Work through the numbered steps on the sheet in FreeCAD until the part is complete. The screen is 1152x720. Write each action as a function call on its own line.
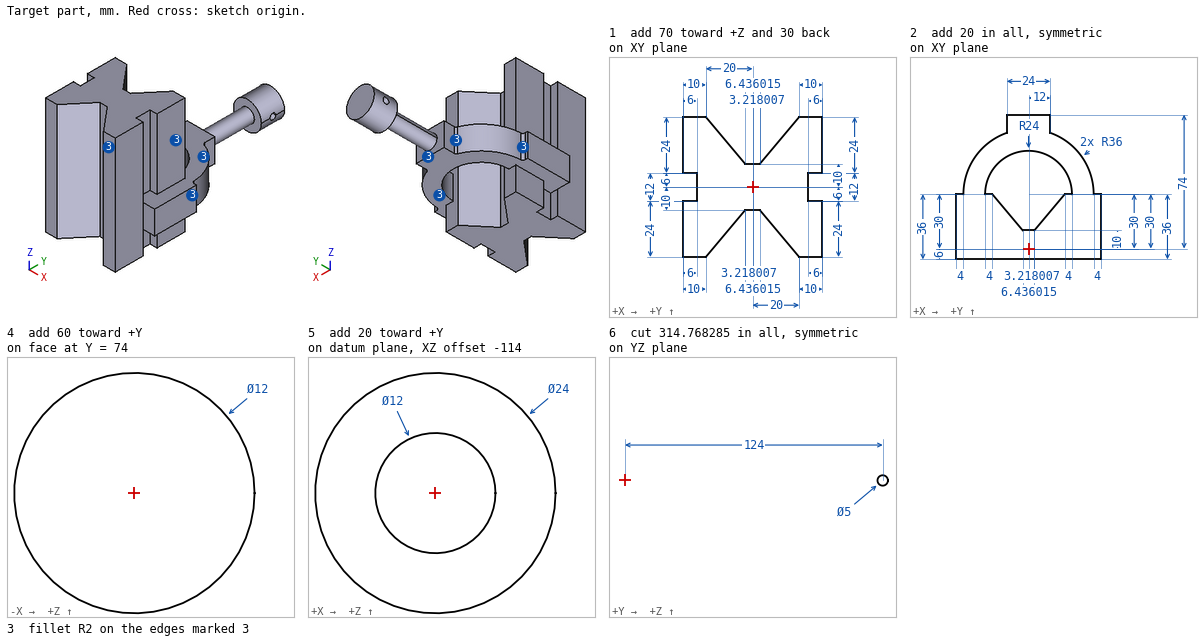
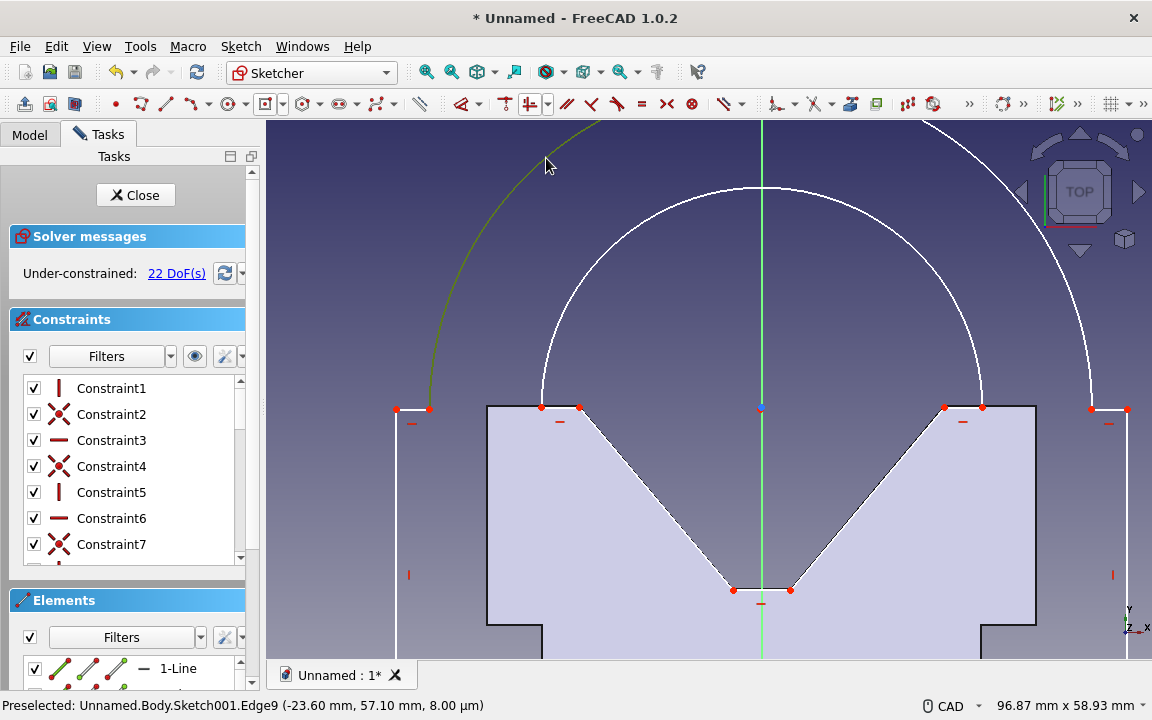
click(891, 230)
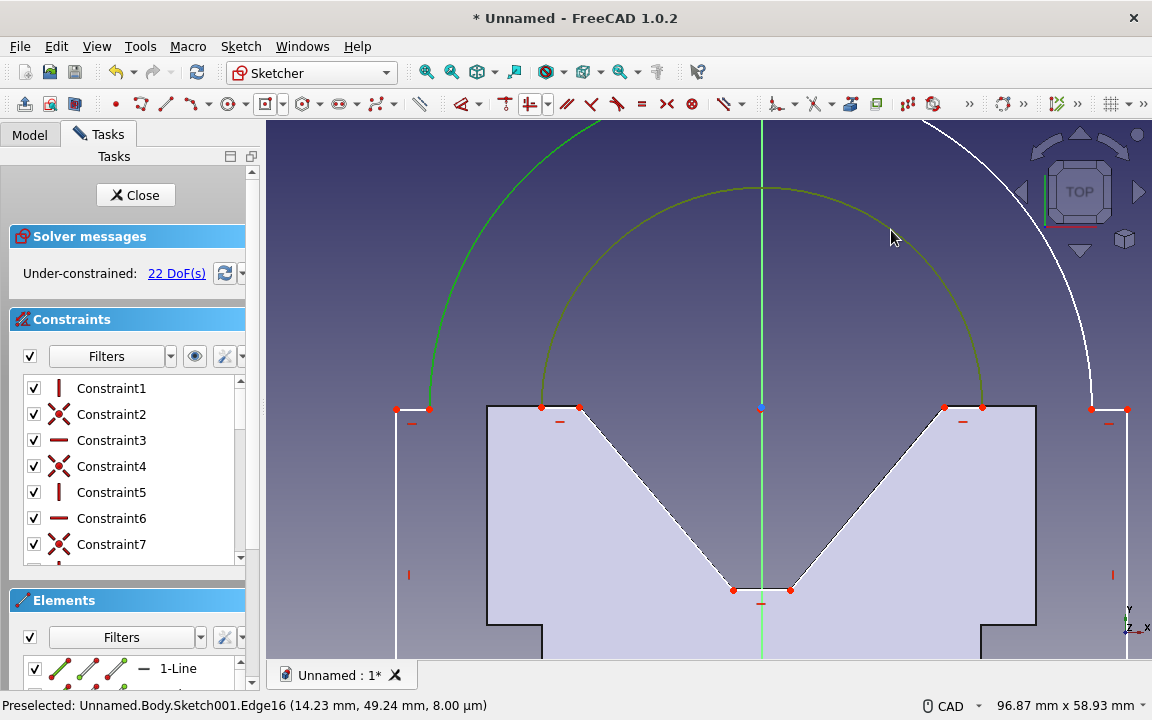
click(505, 104)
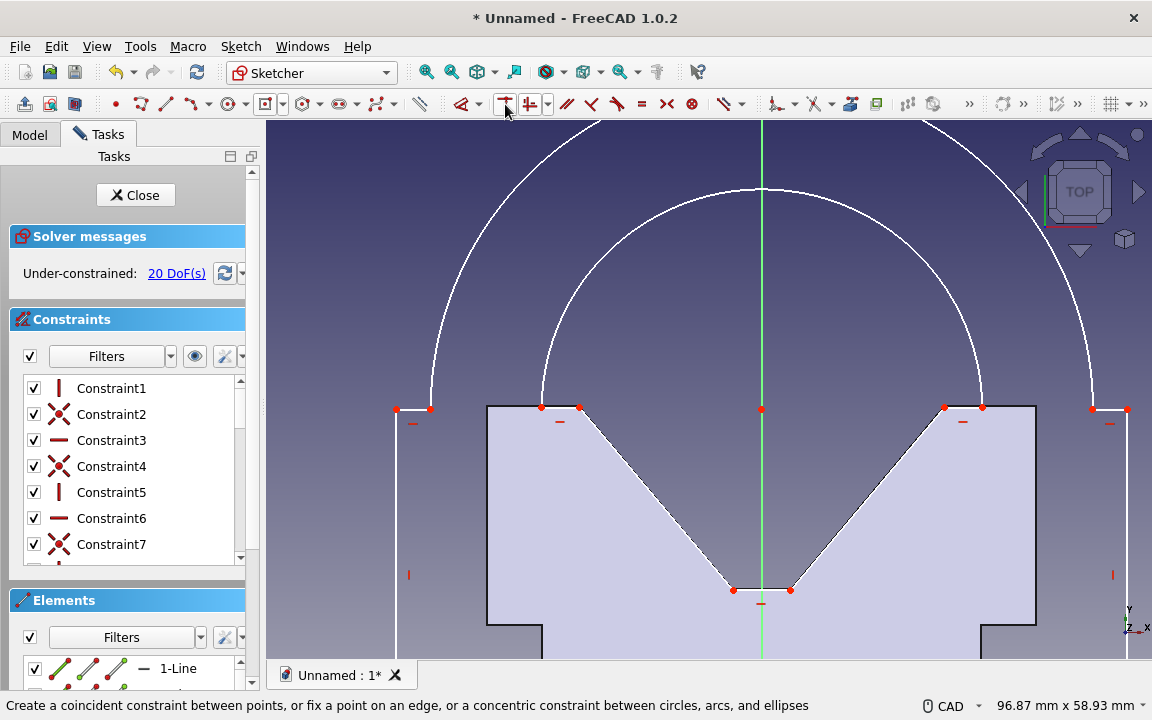
click(546, 158)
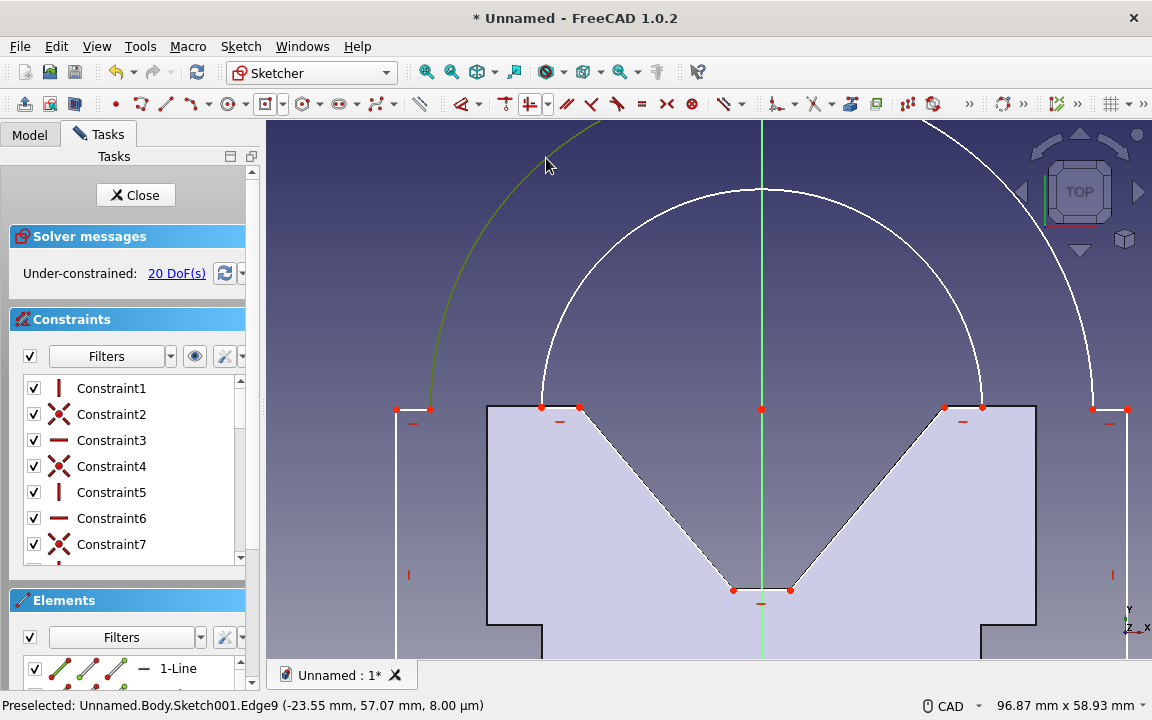
click(977, 158)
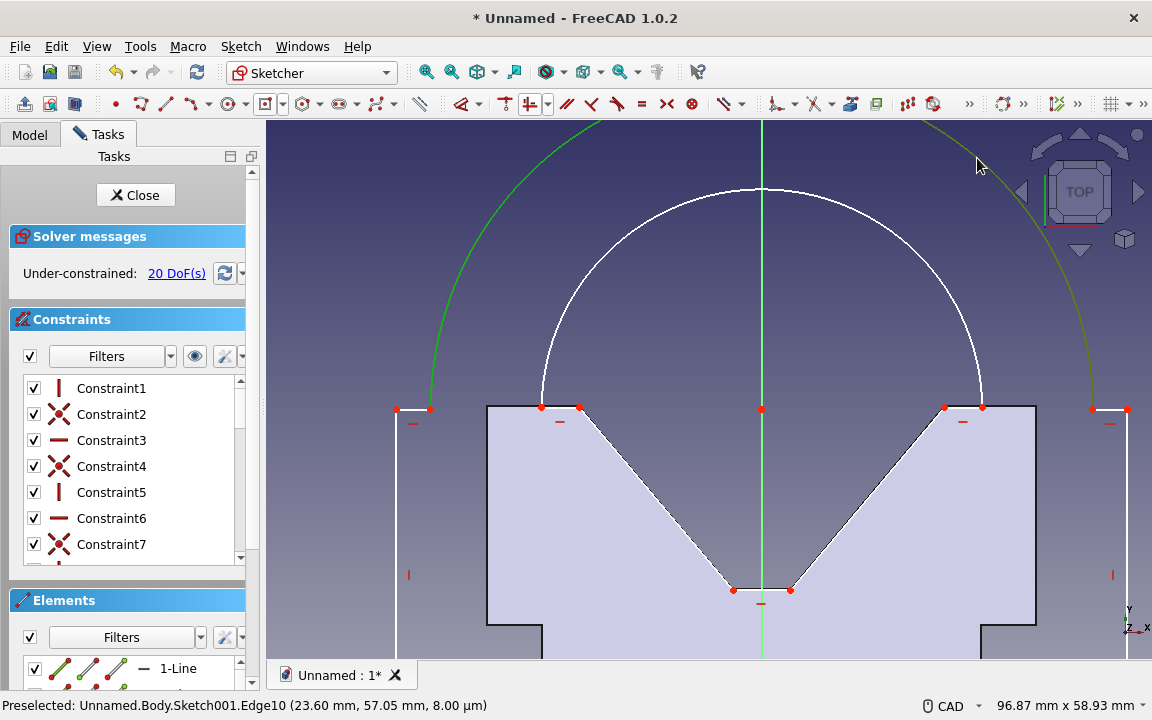
click(642, 104)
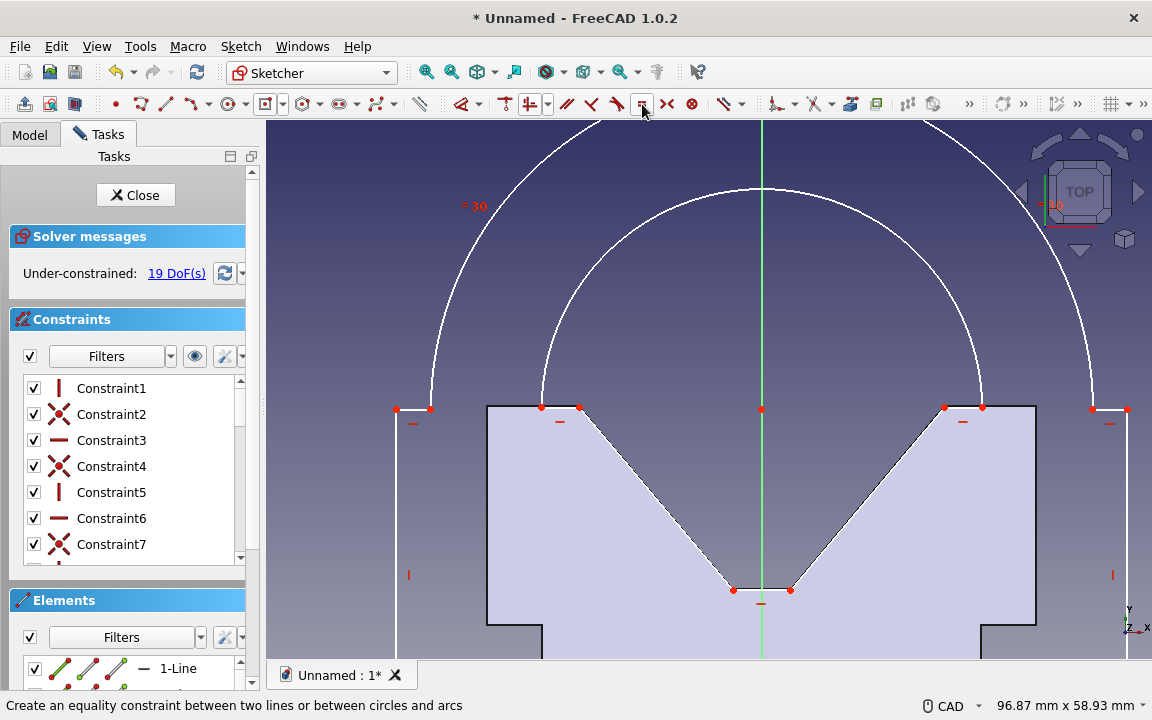
click(762, 409)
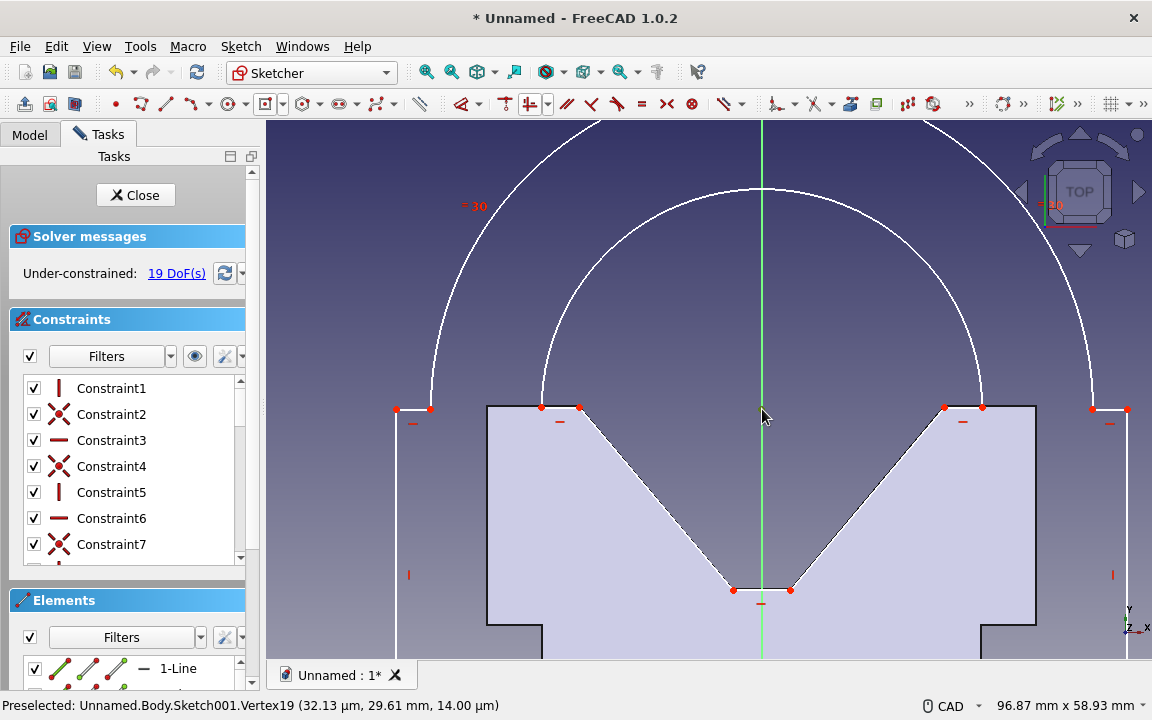
click(762, 528)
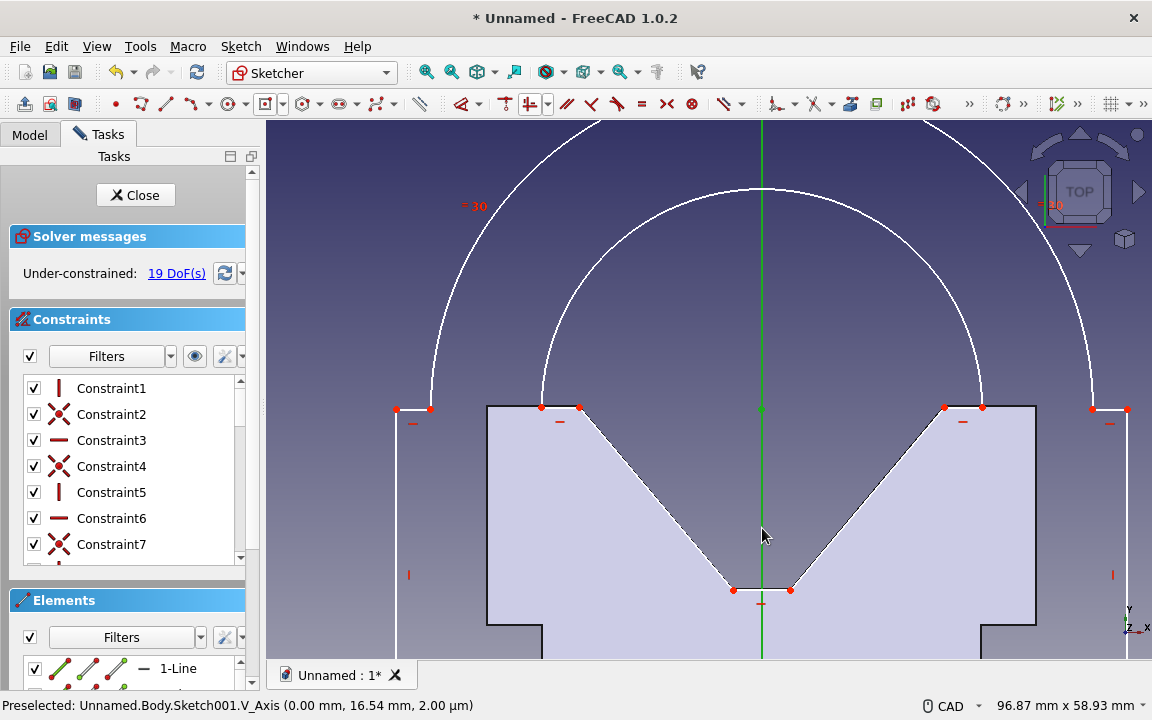
click(505, 104)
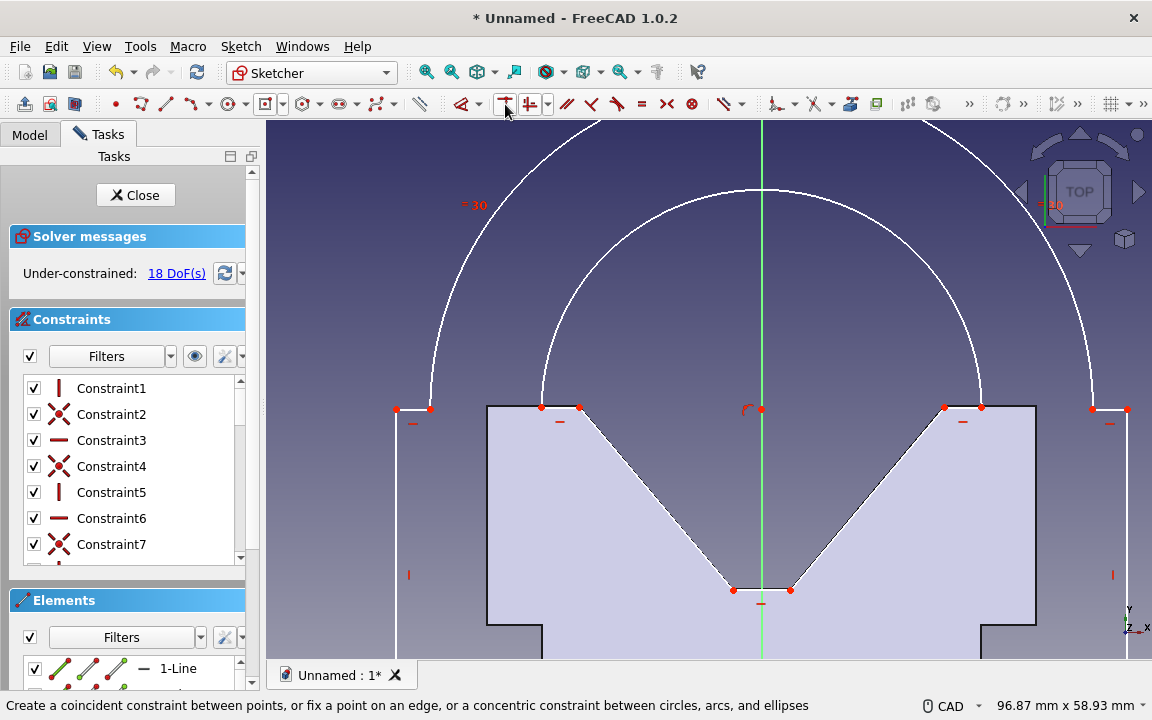
click(460, 104)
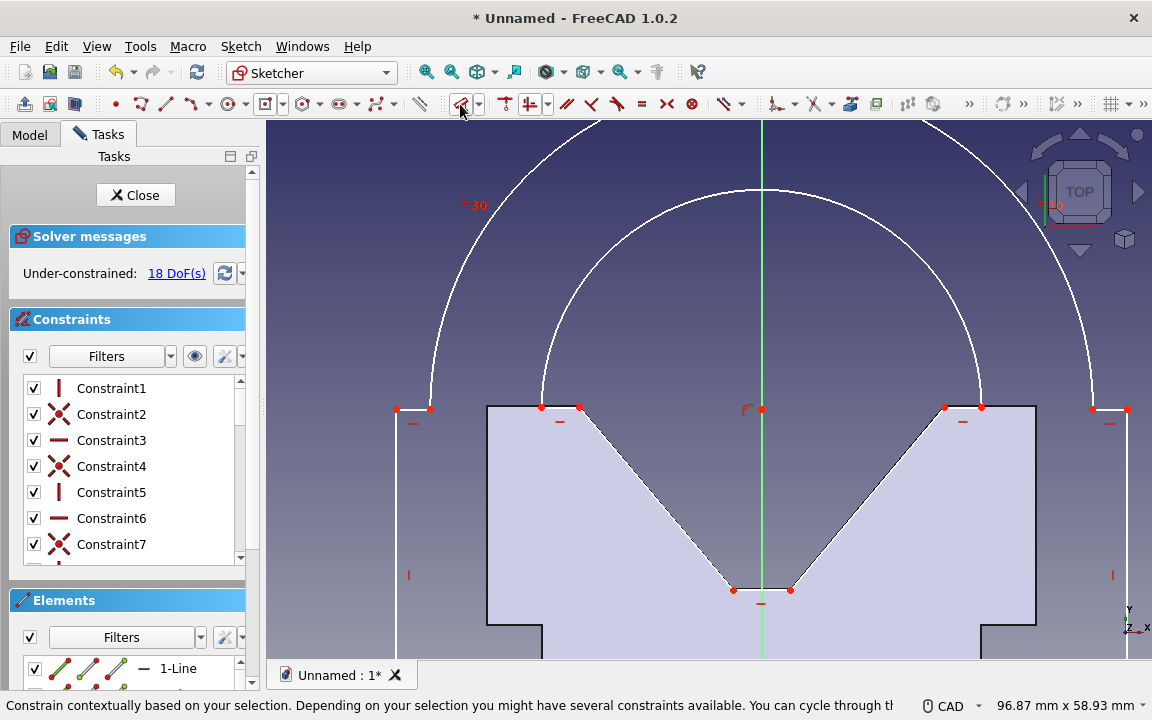
click(546, 158)
click(422, 281)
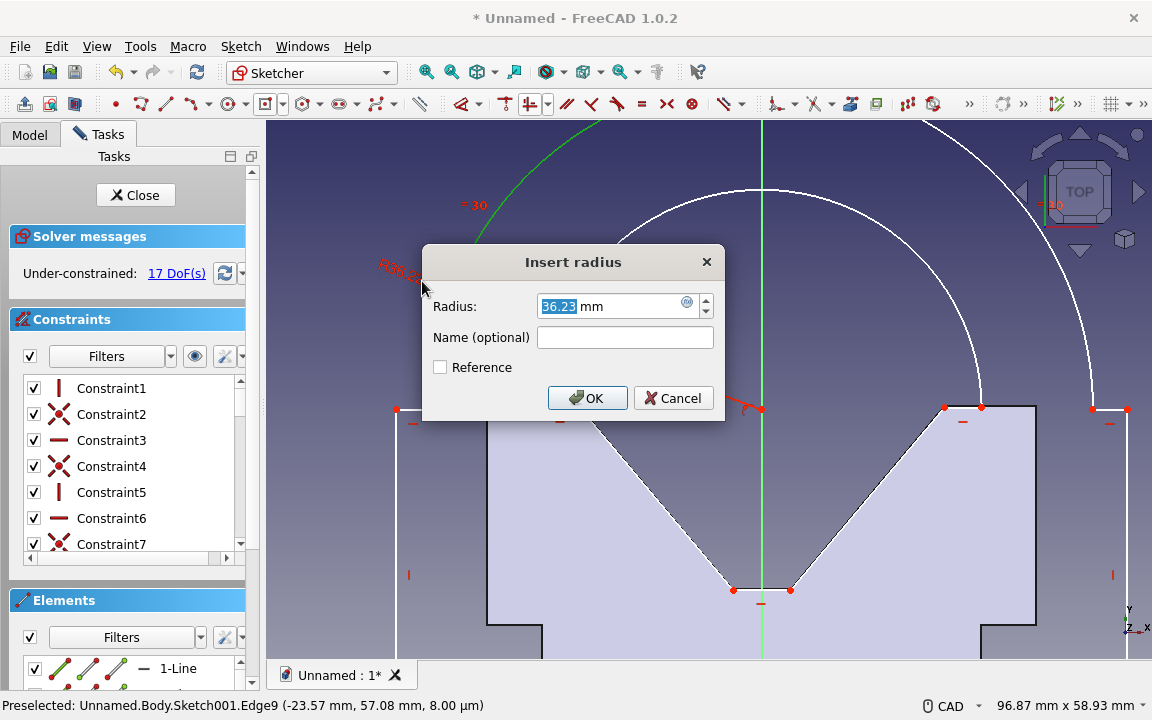
text(36)
key(Return)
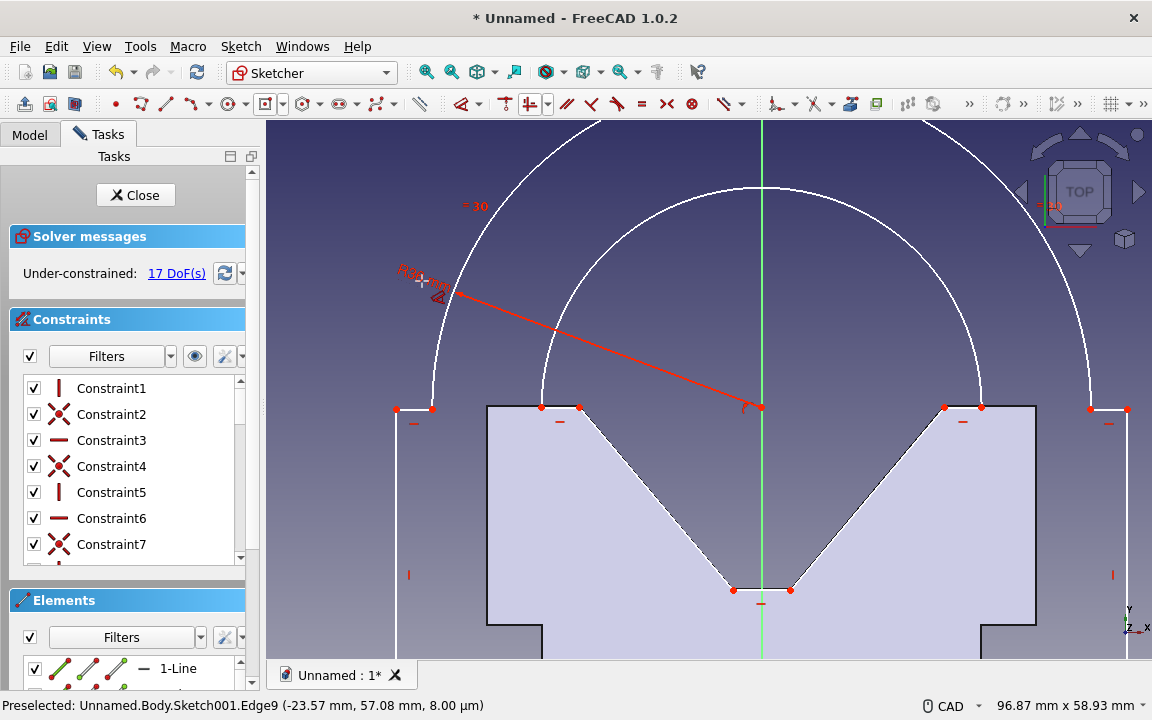
click(891, 230)
click(910, 204)